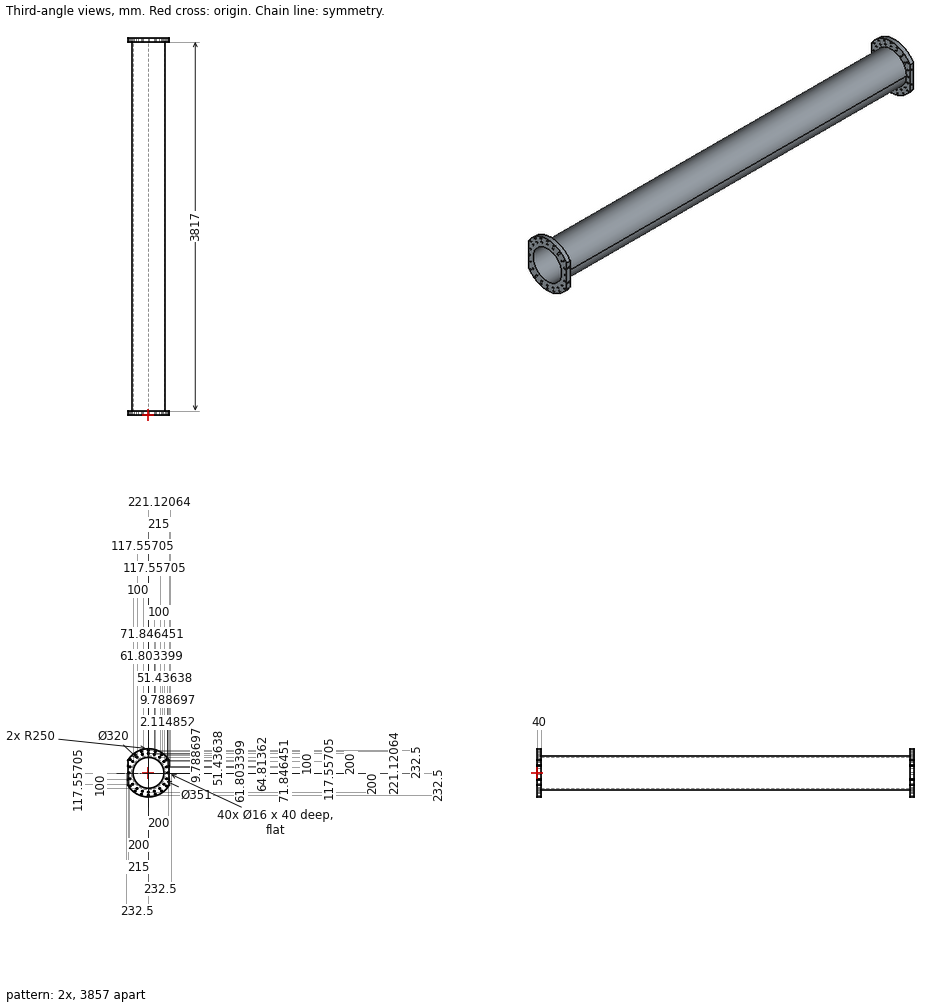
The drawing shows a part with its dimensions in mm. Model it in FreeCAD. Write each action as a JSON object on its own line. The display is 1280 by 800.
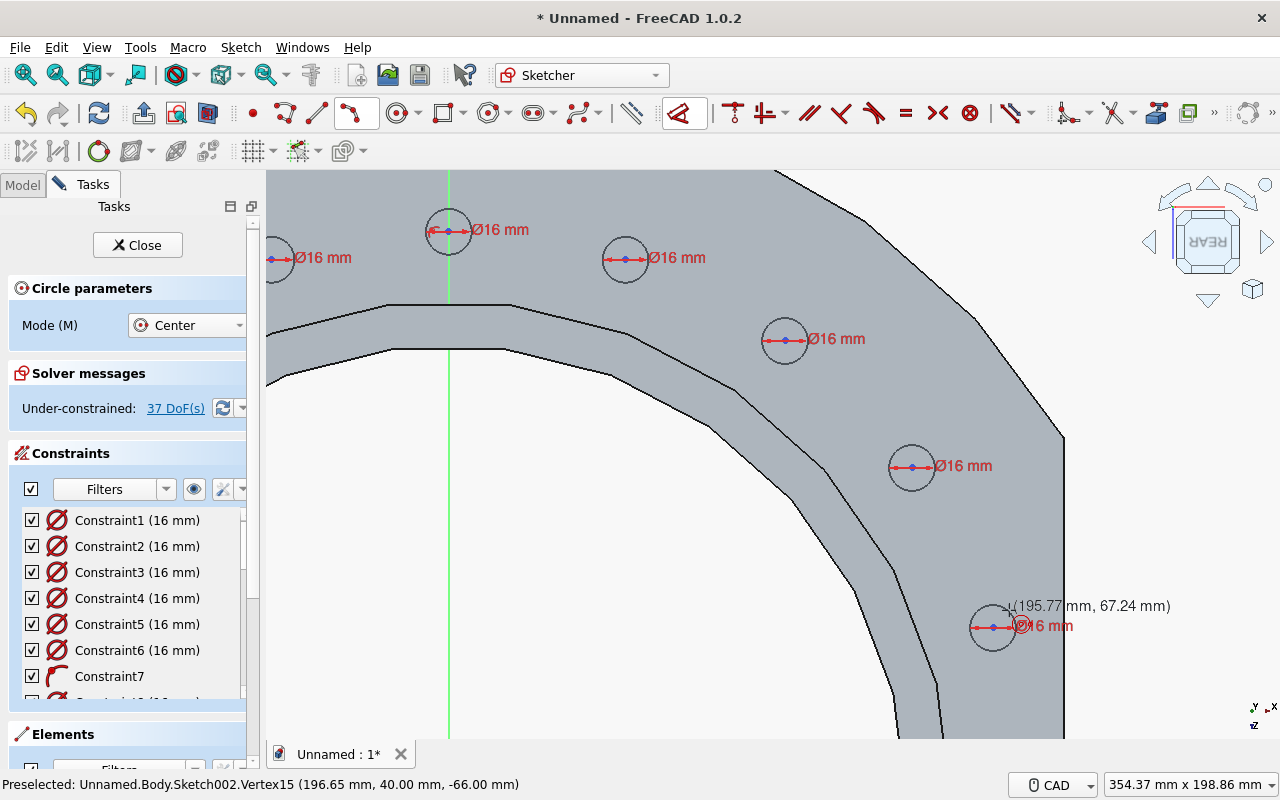
{"action": "scroll", "coordinate": [788, 340], "scroll_direction": "down", "scroll_amount": 7}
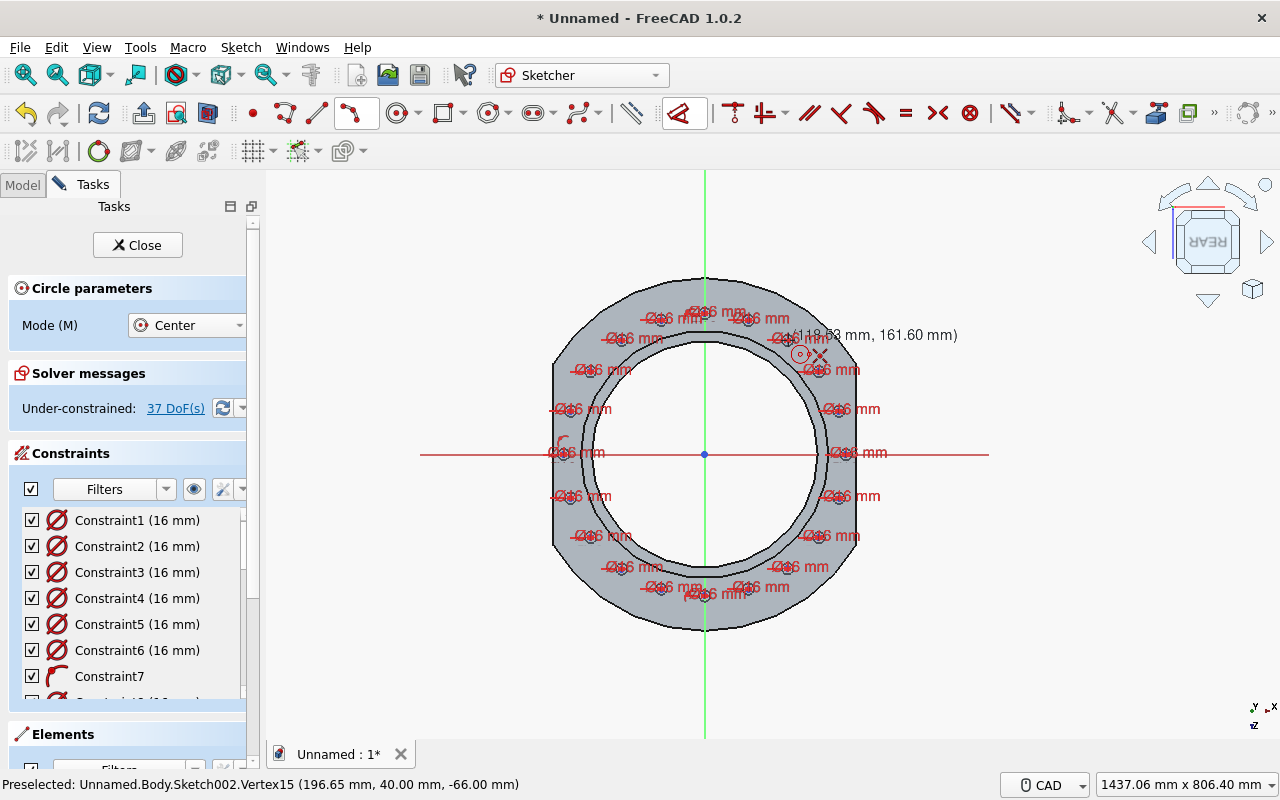
{"action": "scroll", "coordinate": [869, 455], "scroll_direction": "up", "scroll_amount": 7}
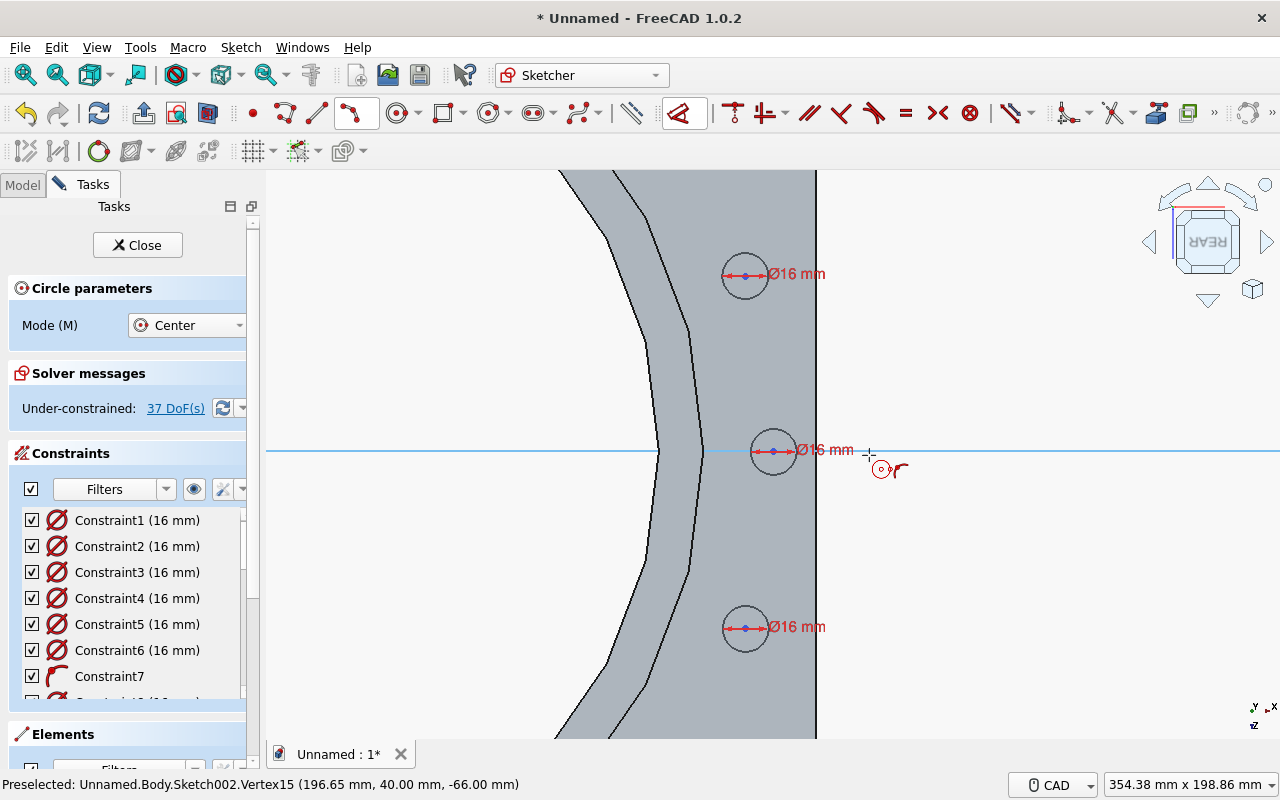
{"action": "left_click", "coordinate": [866, 451]}
{"action": "mouse_move", "coordinate": [883, 435]}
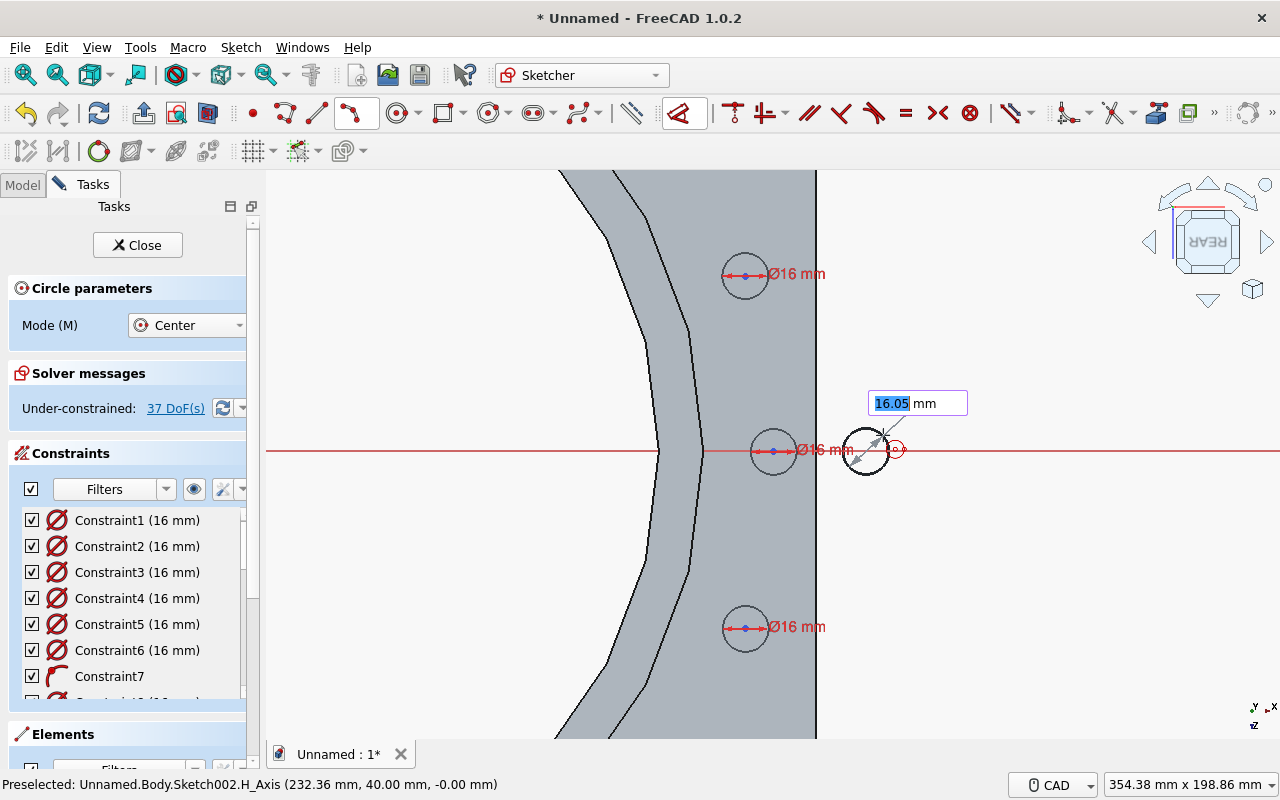
{"action": "type", "text": "16"}
{"action": "key", "text": "Return"}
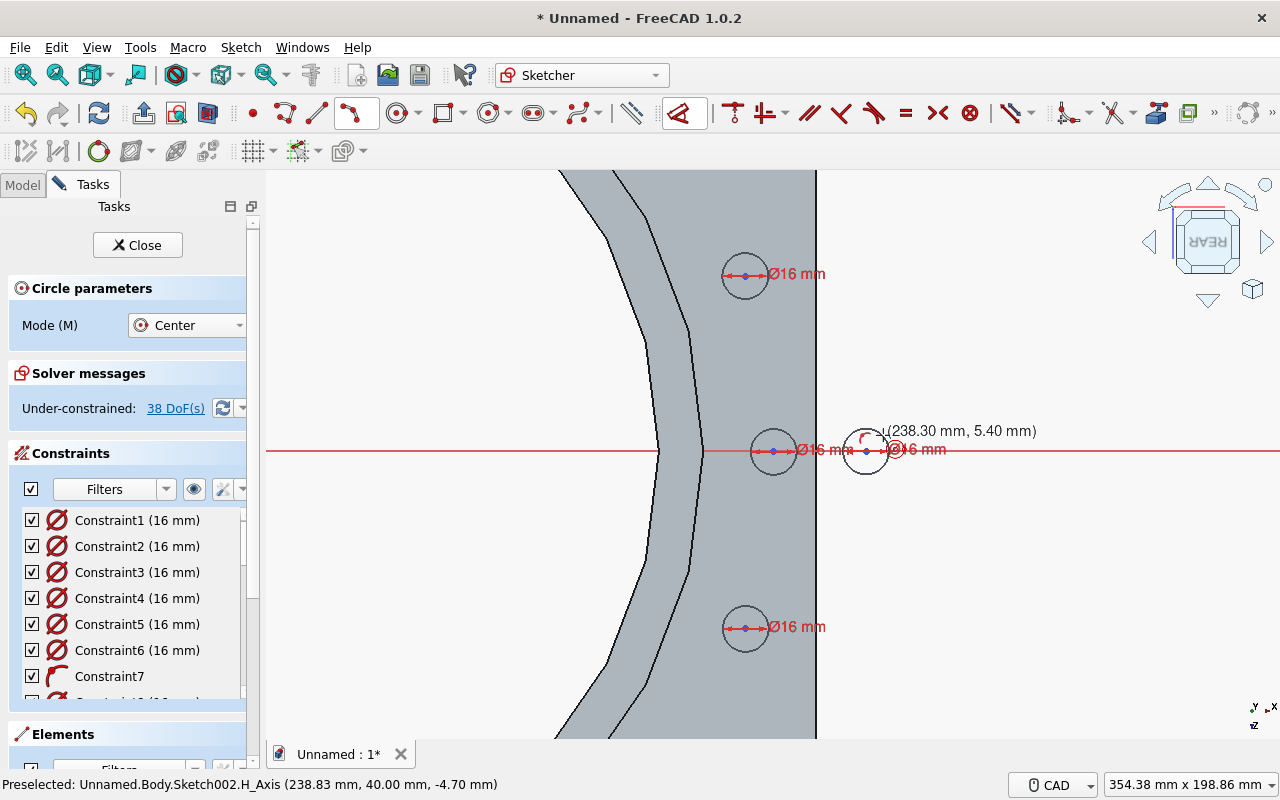
{"action": "left_click", "coordinate": [834, 657]}
{"action": "mouse_move", "coordinate": [850, 641]}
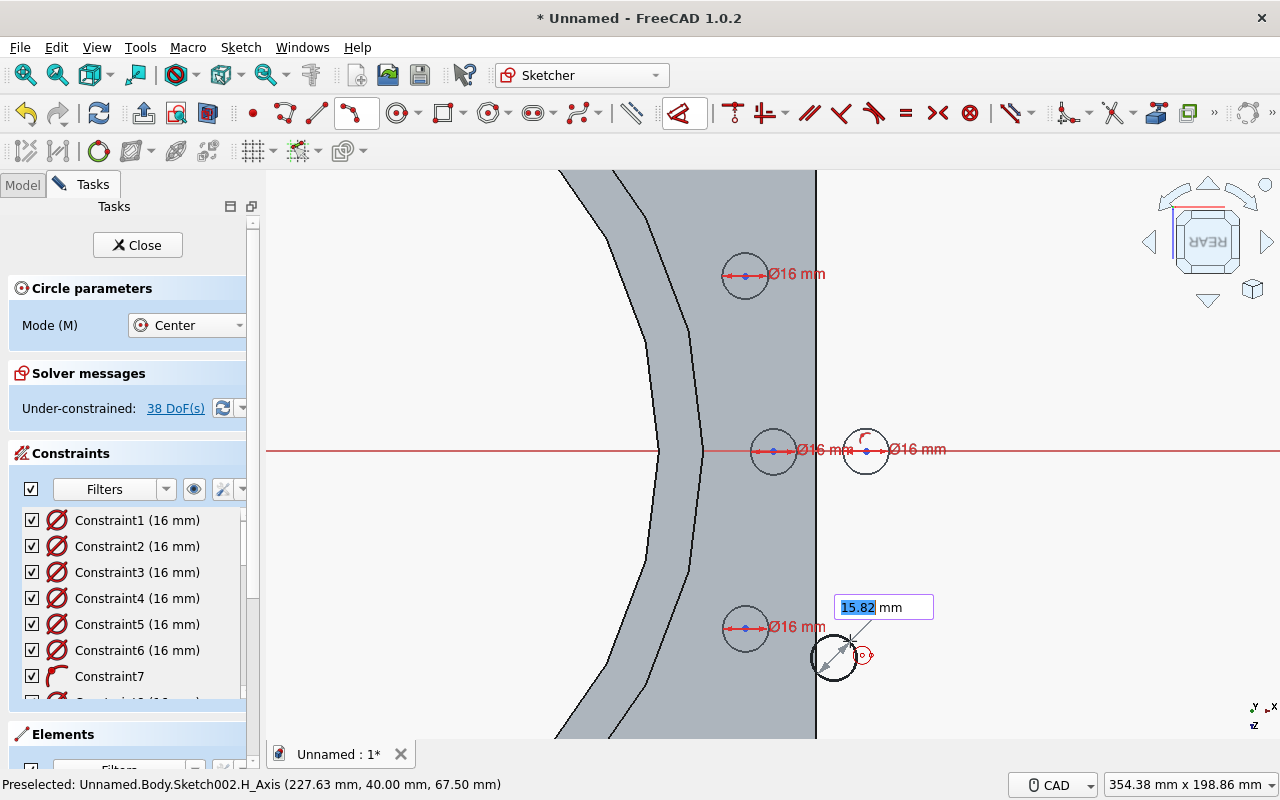
{"action": "type", "text": "16"}
{"action": "key", "text": "Return"}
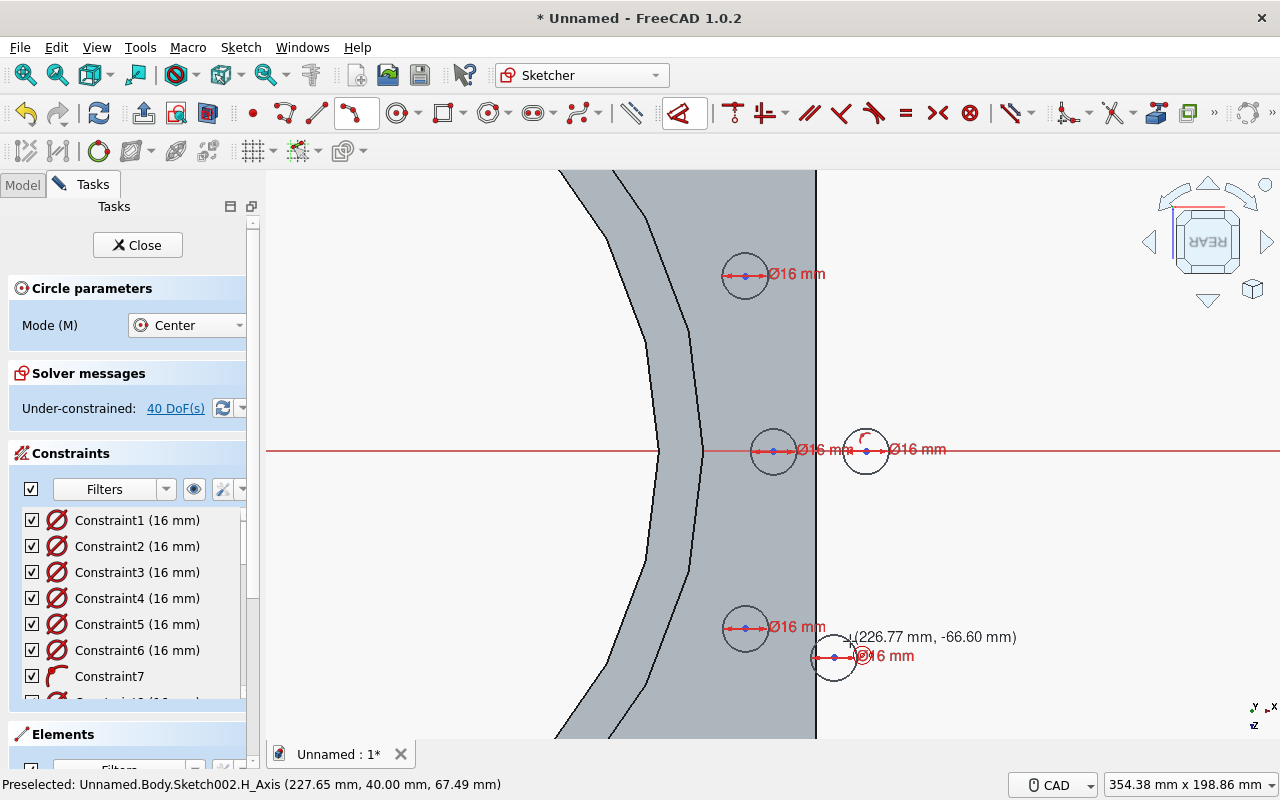
{"action": "scroll", "coordinate": [869, 456], "scroll_direction": "down", "scroll_amount": 7}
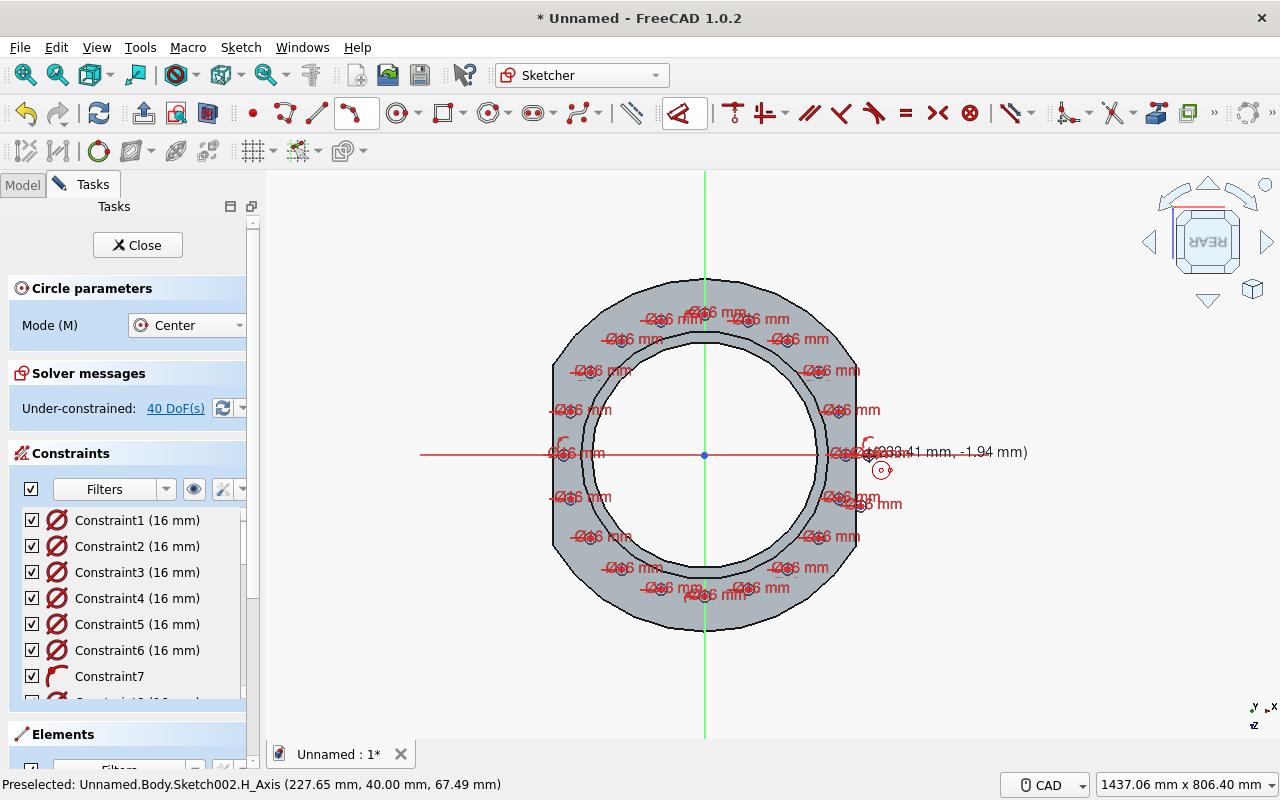
{"action": "scroll", "coordinate": [837, 552], "scroll_direction": "up", "scroll_amount": 7}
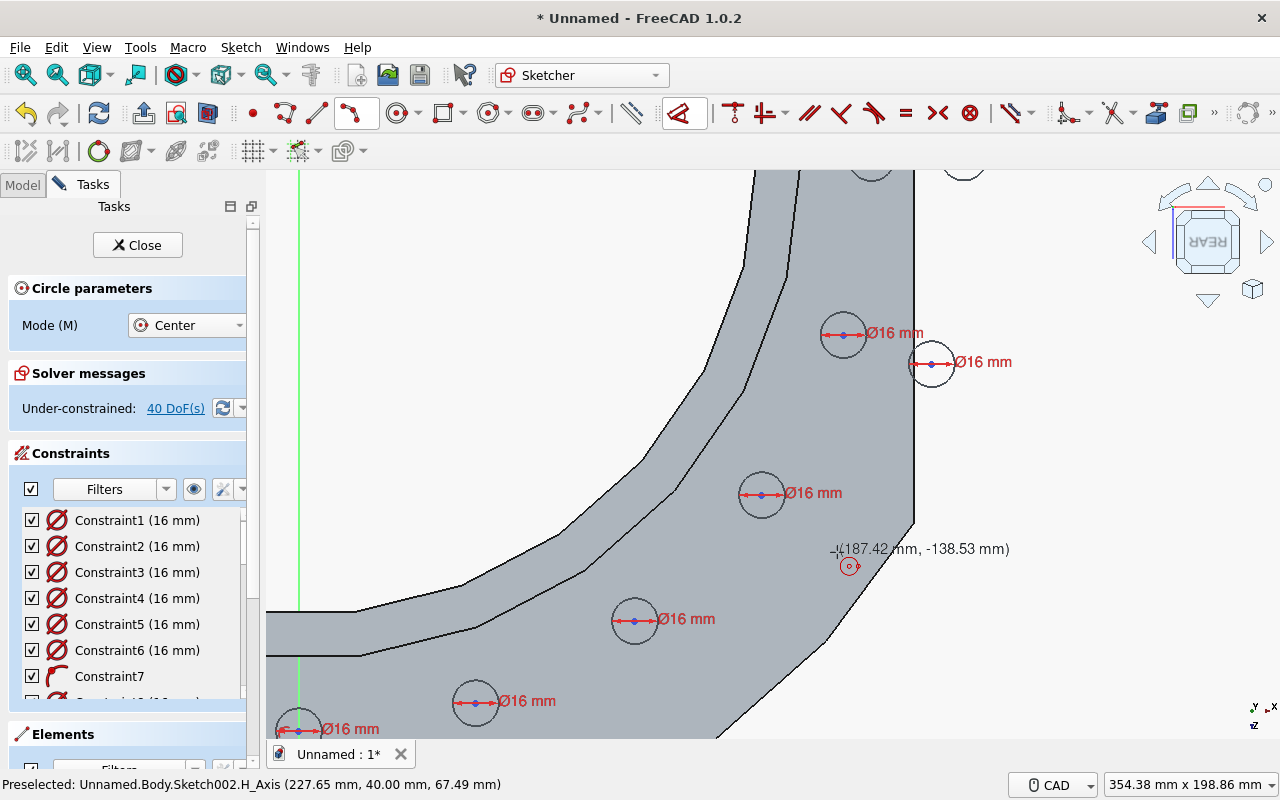
{"action": "left_click", "coordinate": [837, 549]}
{"action": "mouse_move", "coordinate": [853, 532]}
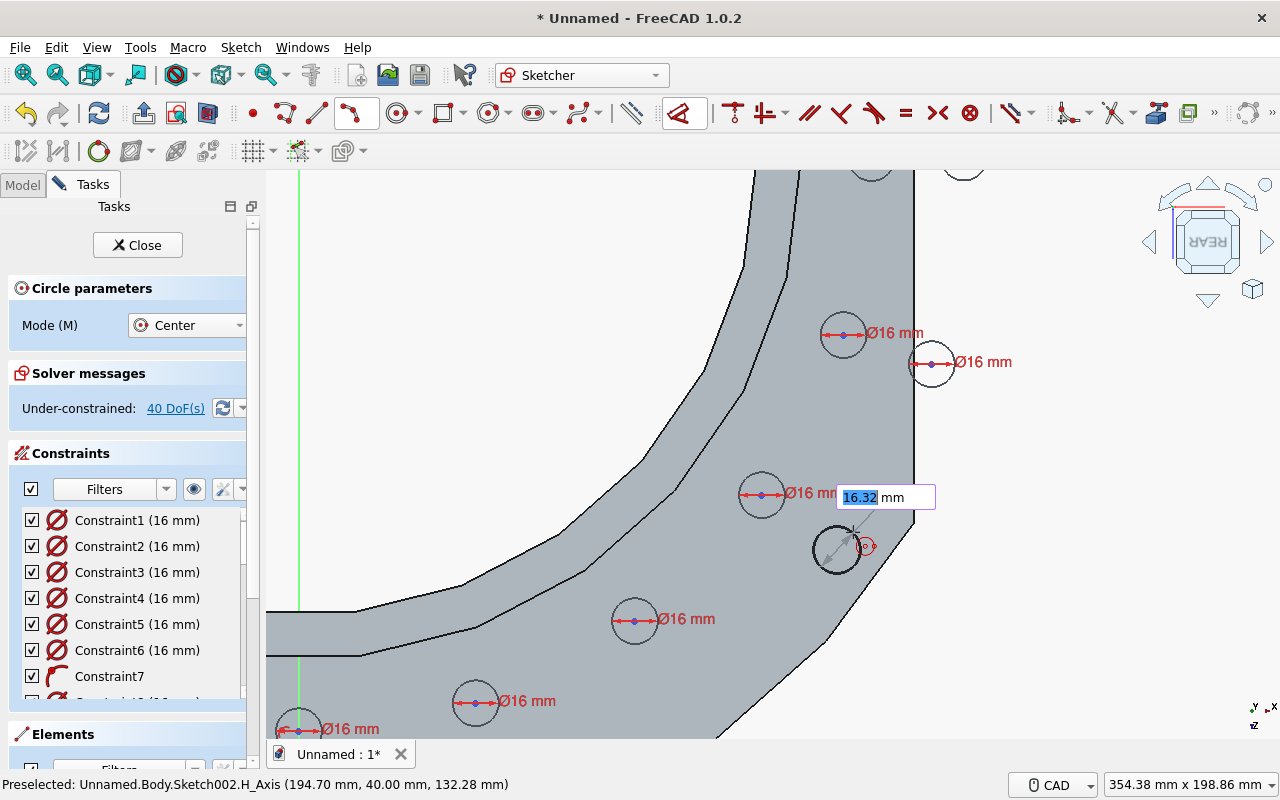
{"action": "type", "text": "16"}
{"action": "key", "text": "Return"}